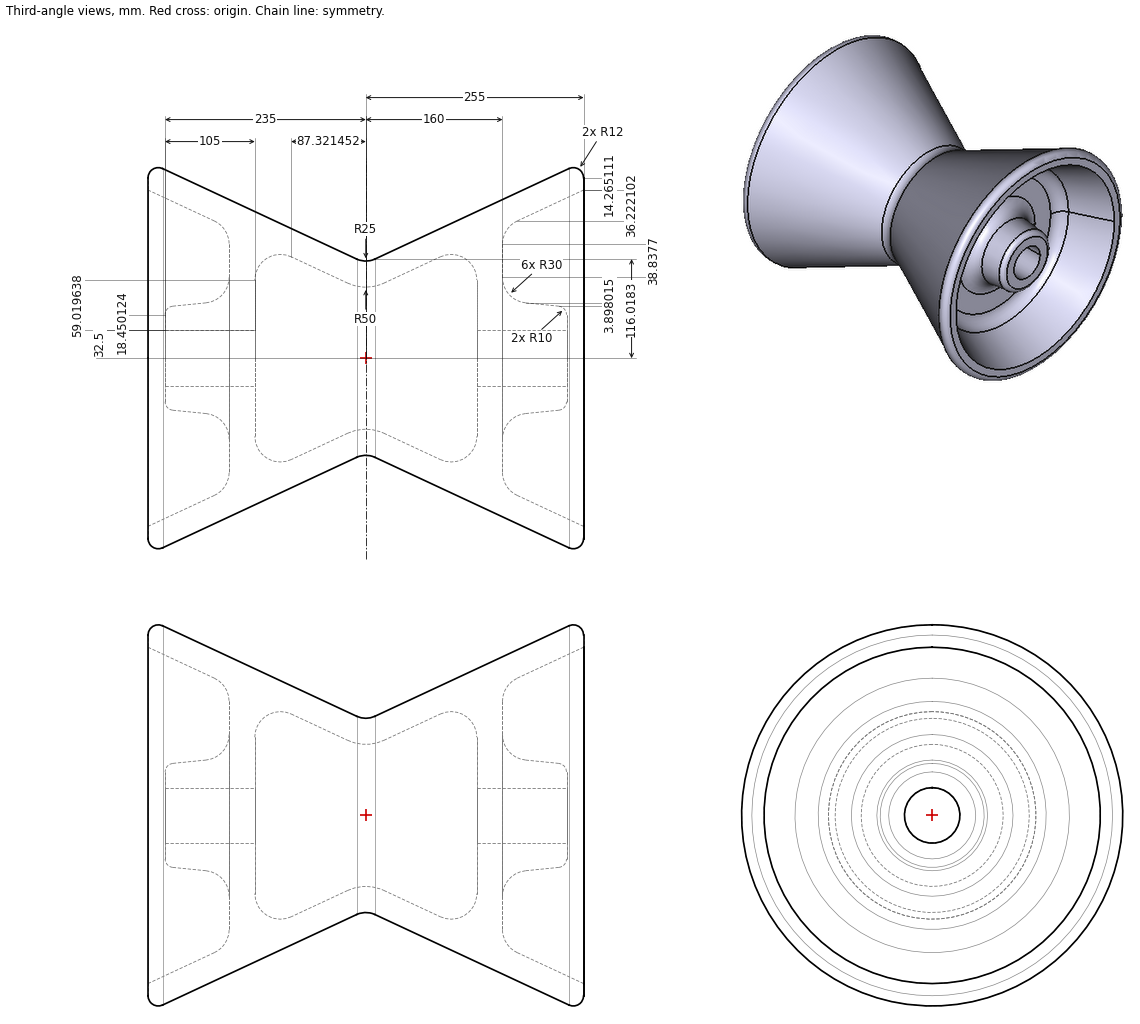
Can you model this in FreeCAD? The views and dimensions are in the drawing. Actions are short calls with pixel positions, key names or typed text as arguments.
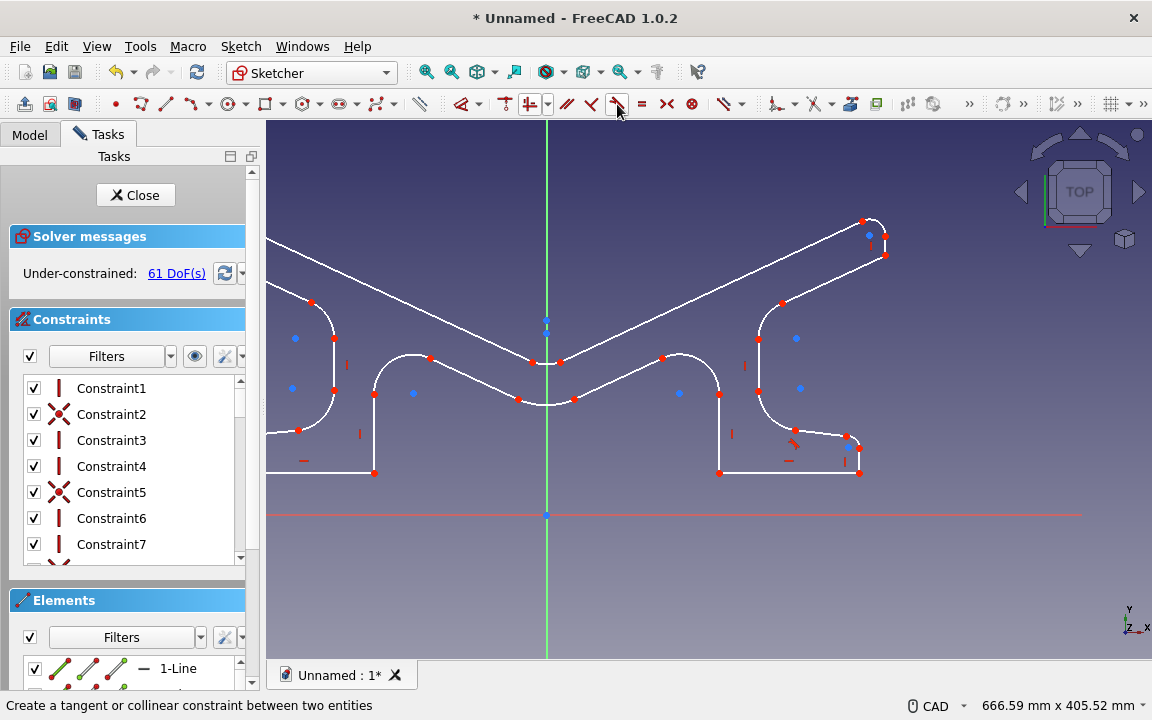
click(831, 434)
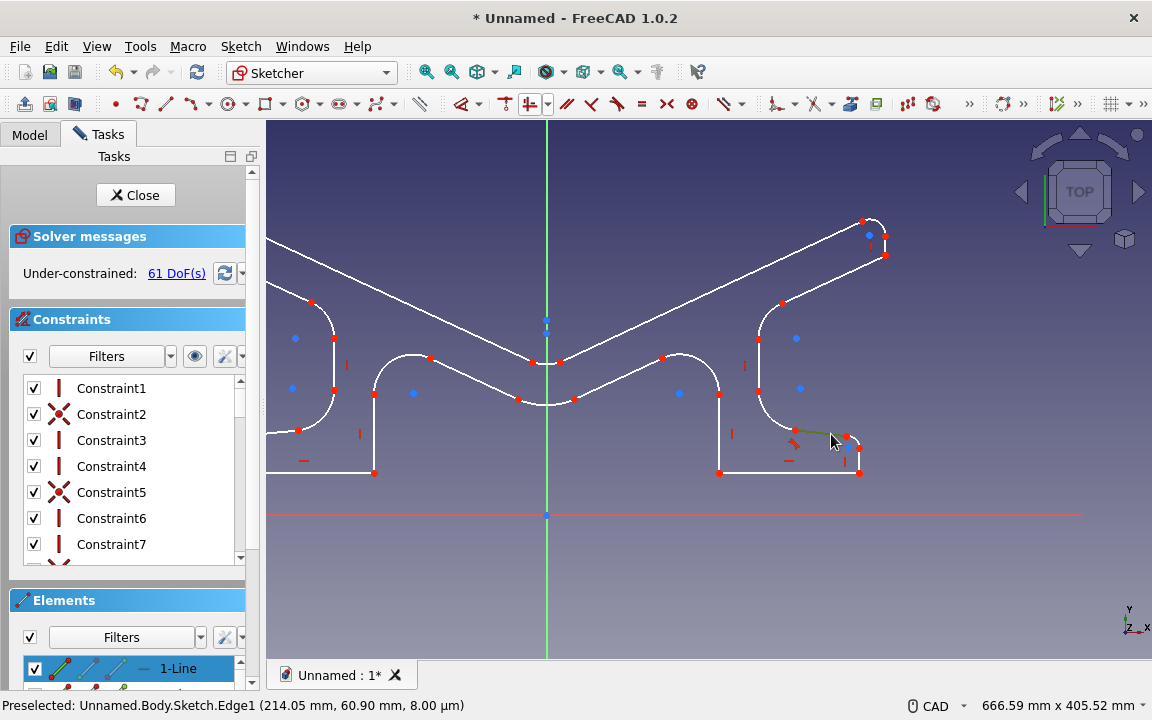
scroll(856, 439, up, 2)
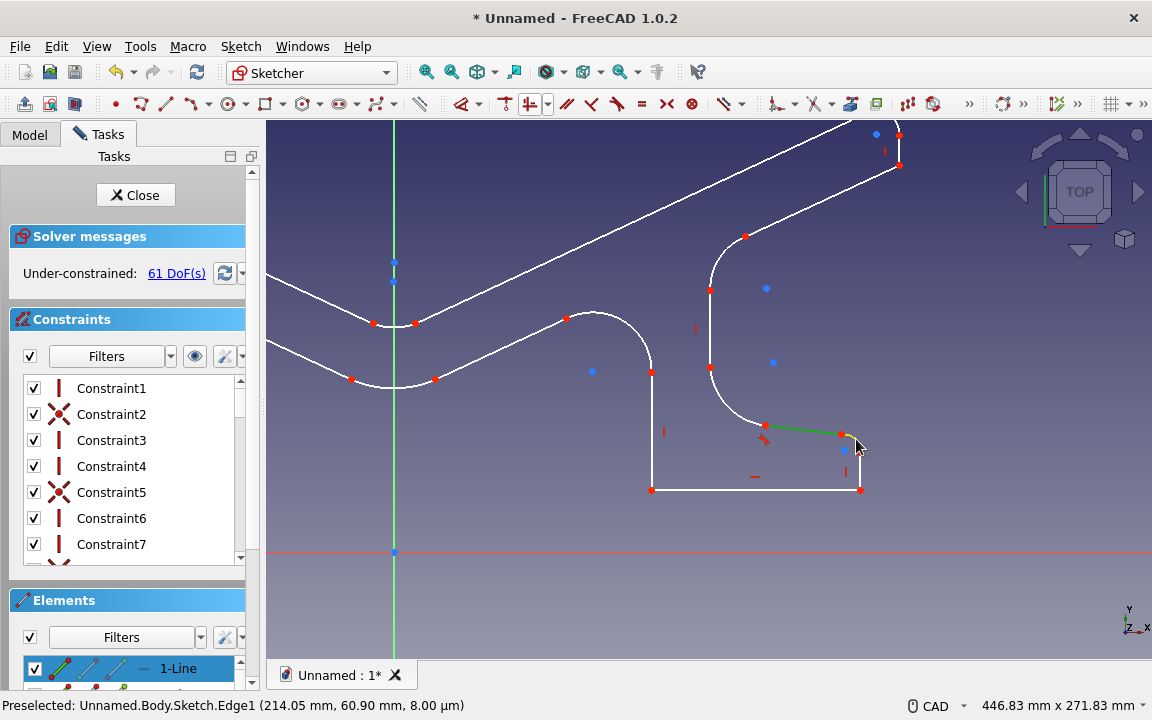
click(855, 439)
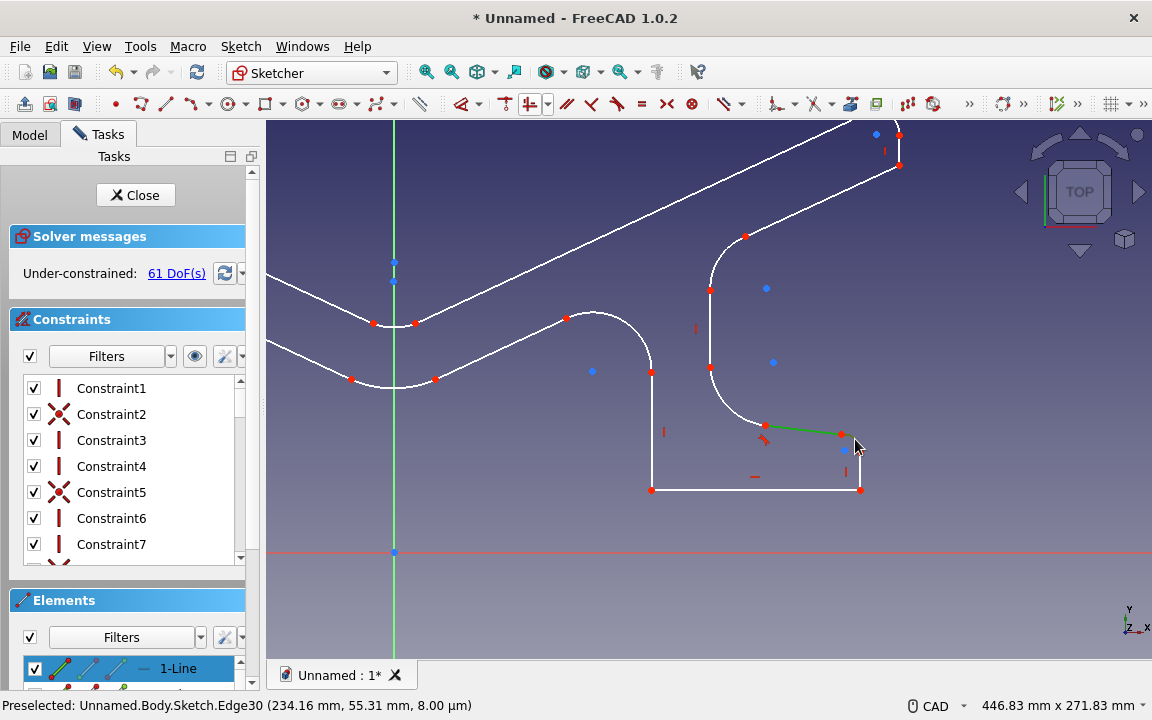
click(617, 104)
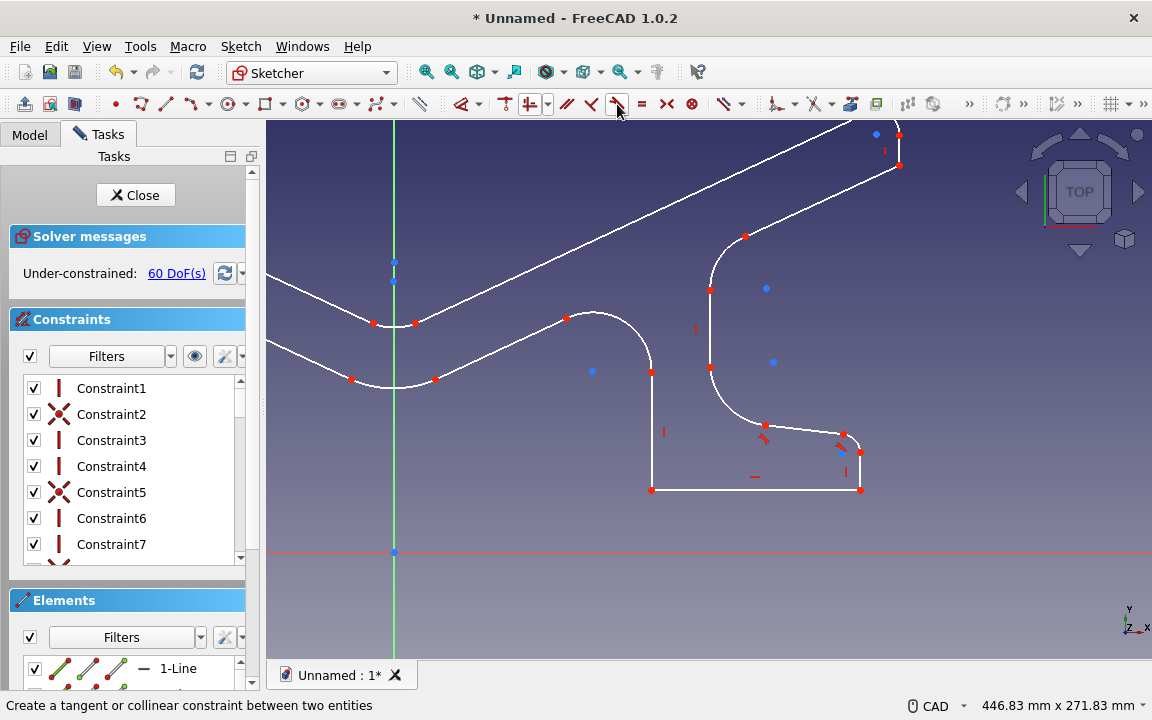
click(710, 345)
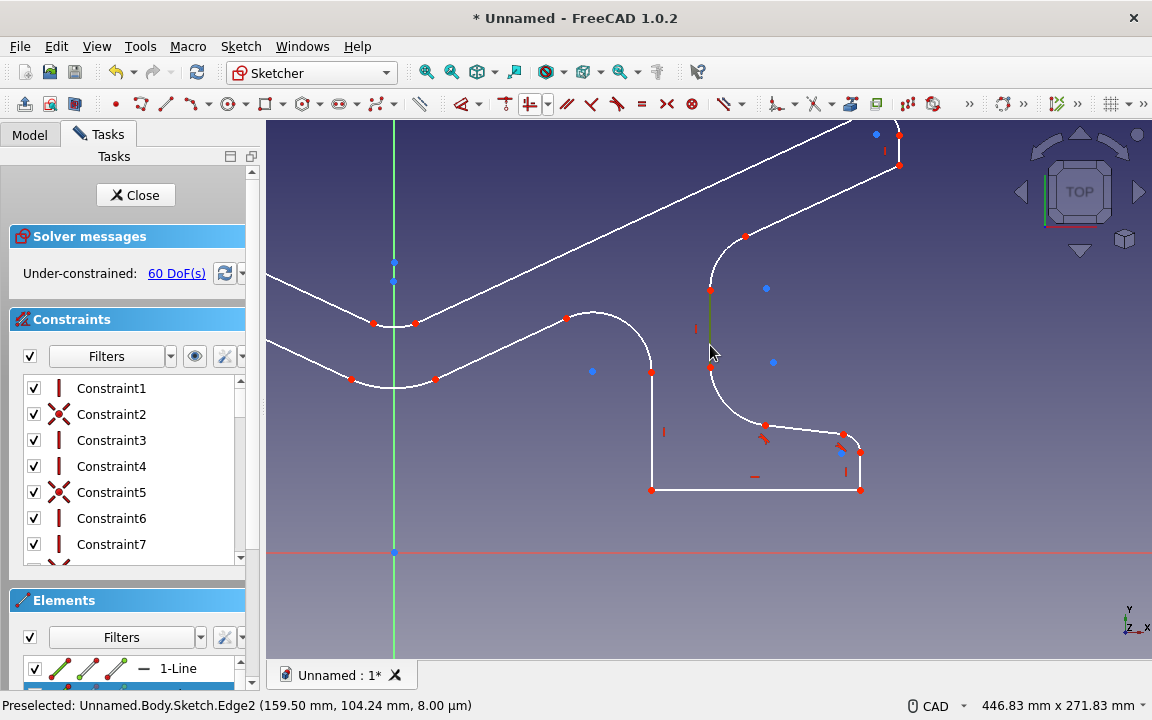
click(718, 393)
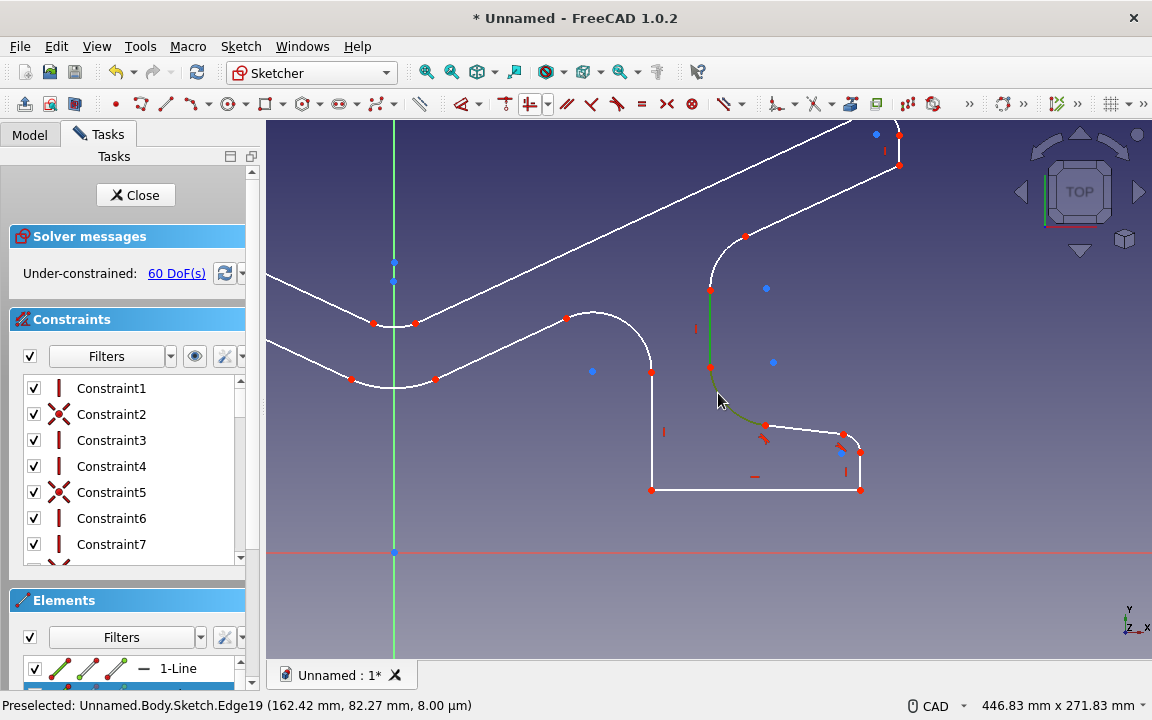
key(t)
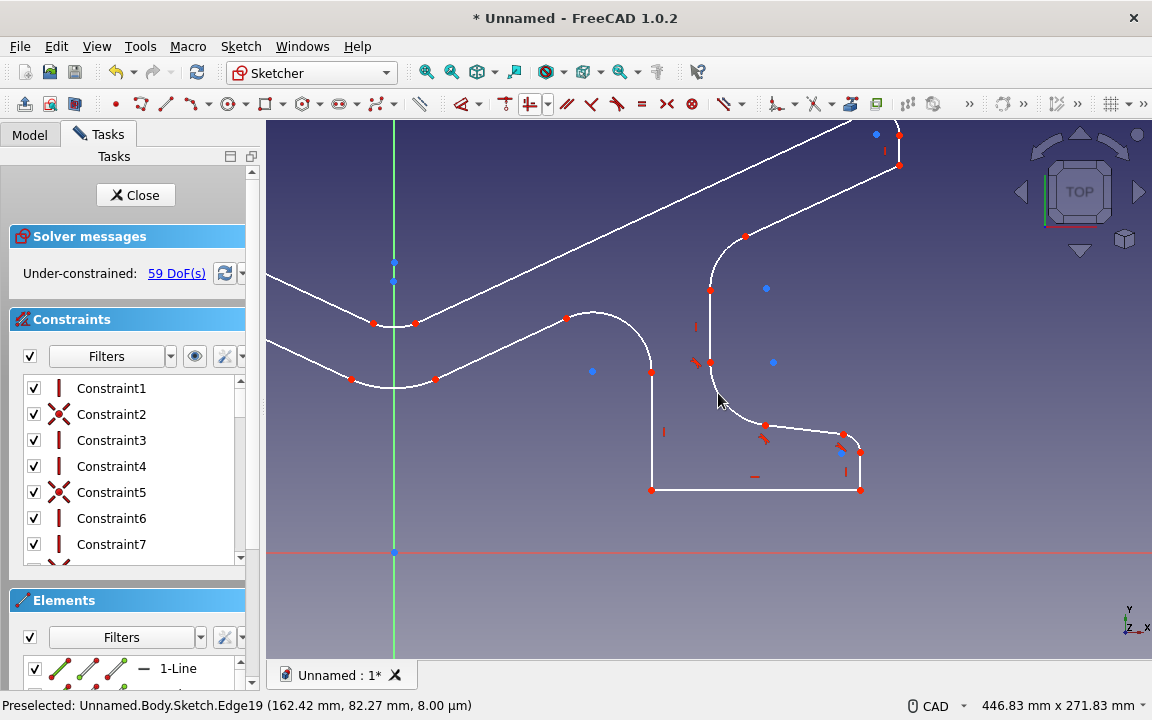
click(710, 341)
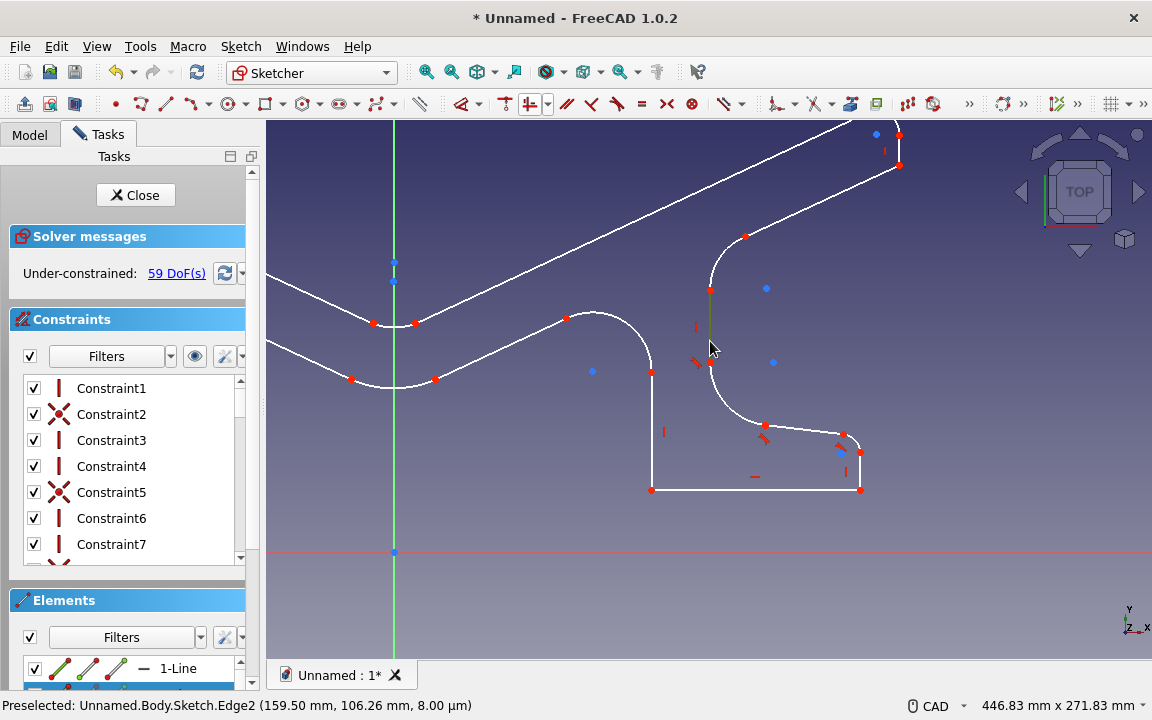
click(729, 247)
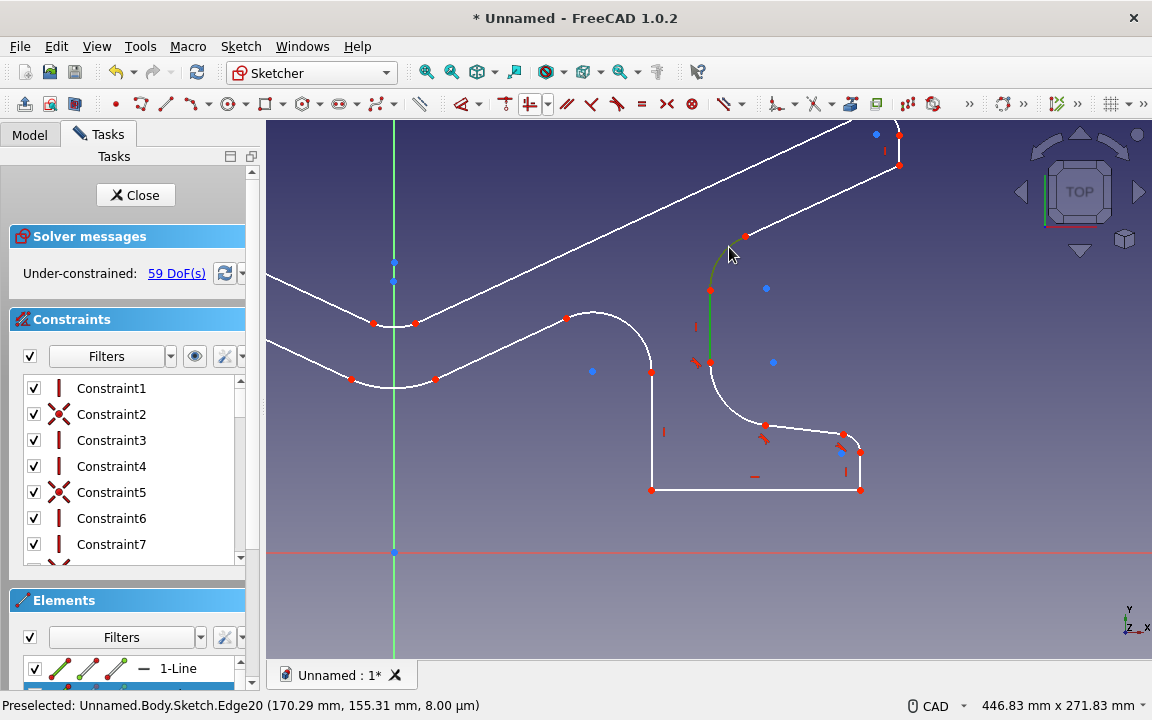
key(t)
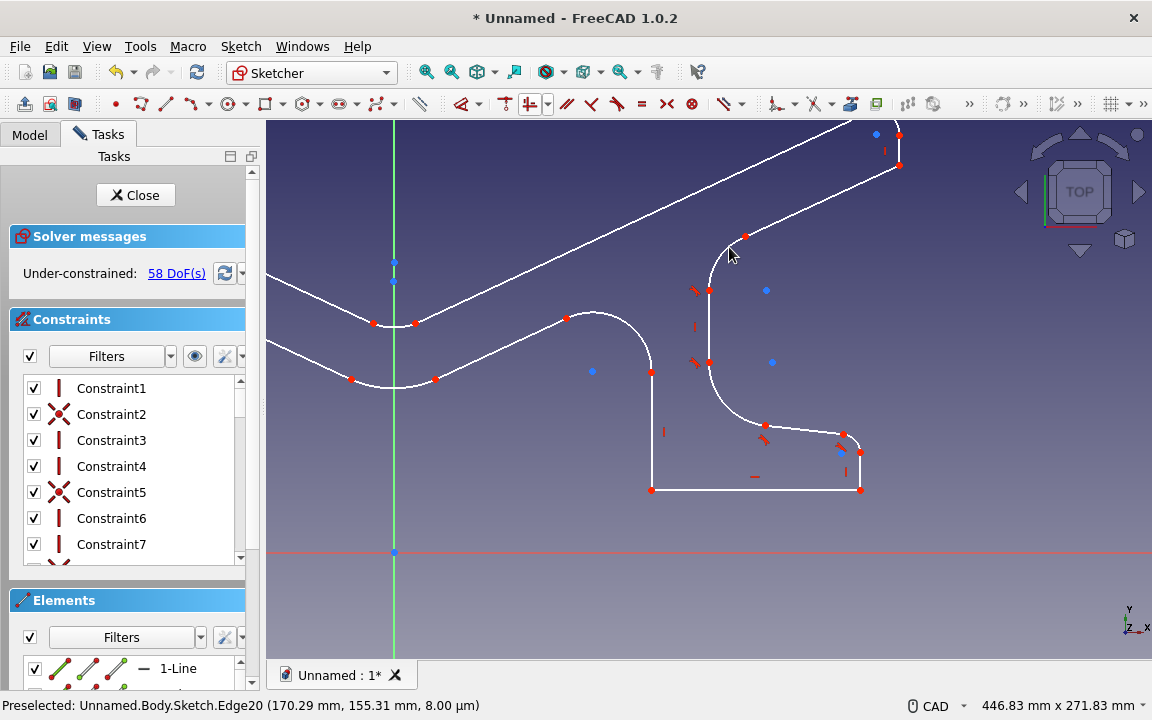
click(792, 215)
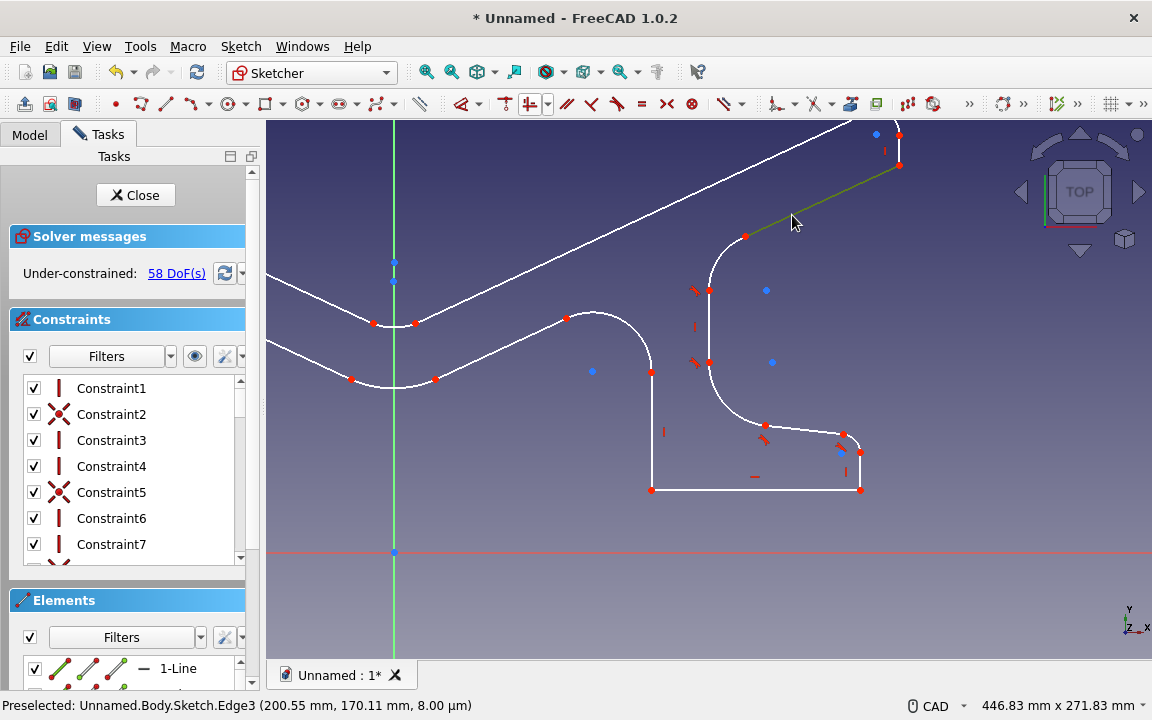
click(728, 247)